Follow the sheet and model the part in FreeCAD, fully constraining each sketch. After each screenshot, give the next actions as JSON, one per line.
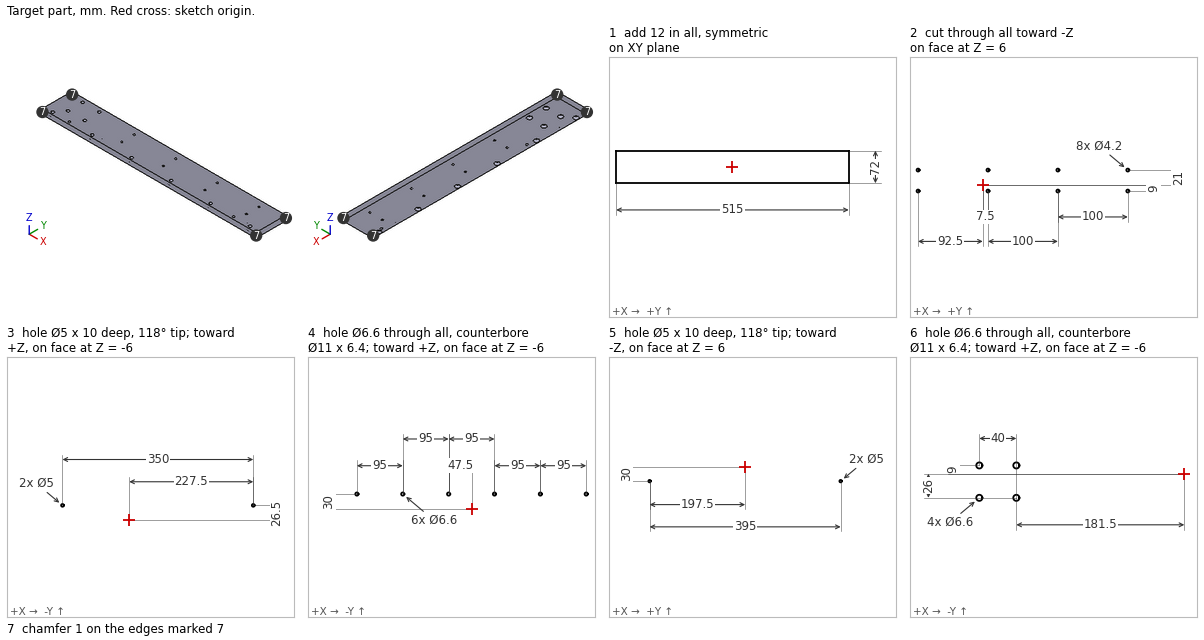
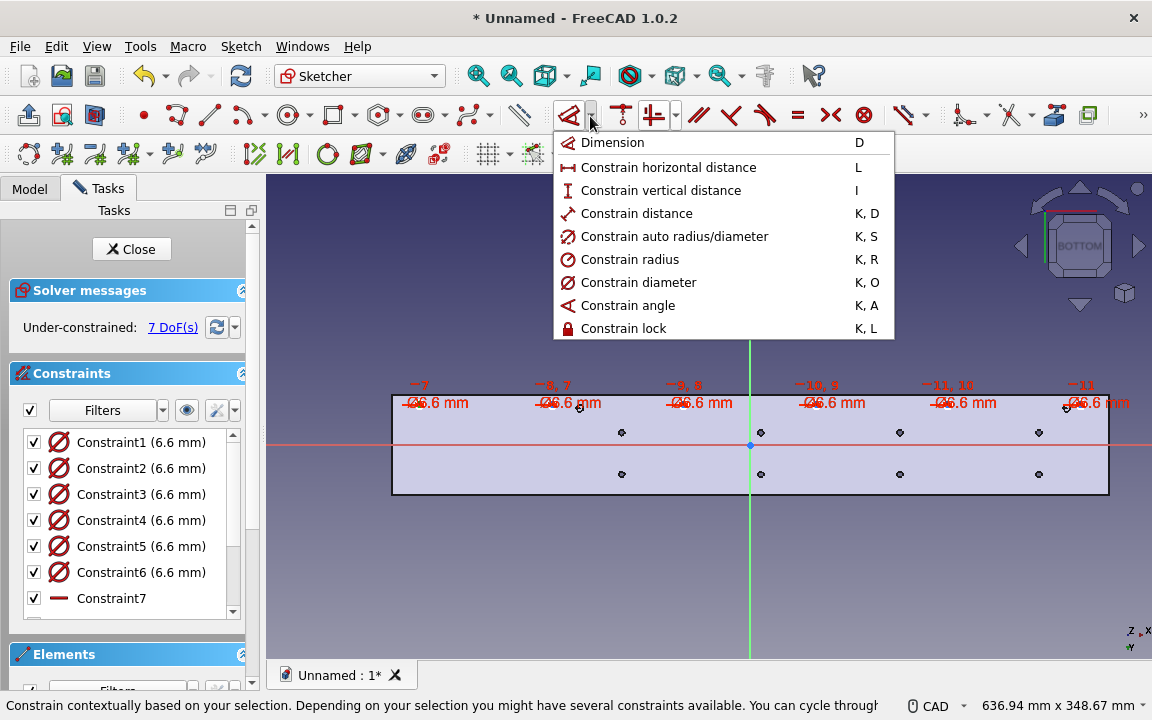
{"action": "left_click", "coordinate": [724, 190]}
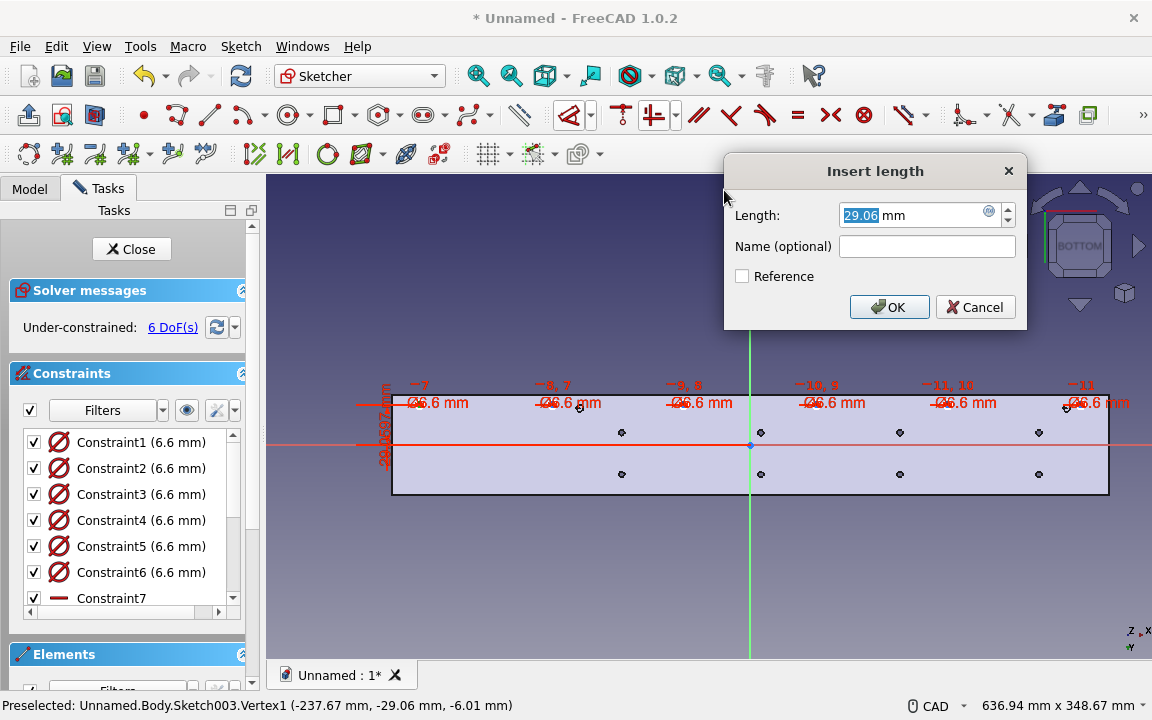
{"action": "type", "text": "30"}
{"action": "key", "text": "Return"}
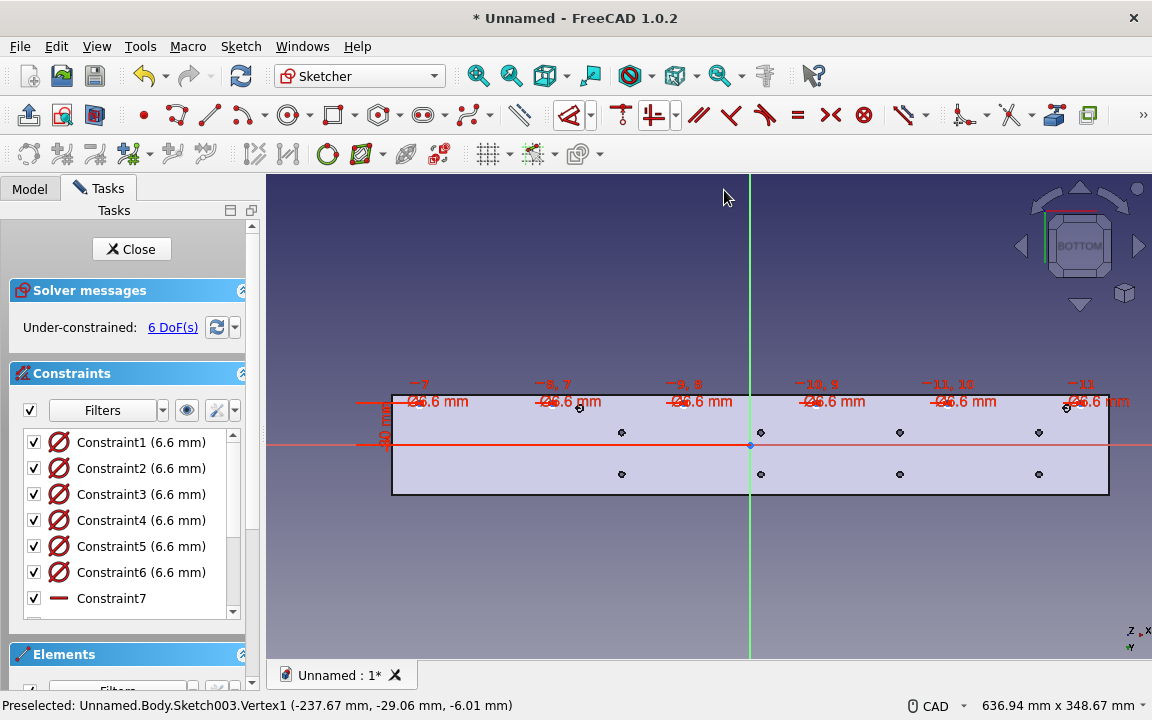
{"action": "left_click", "coordinate": [420, 403]}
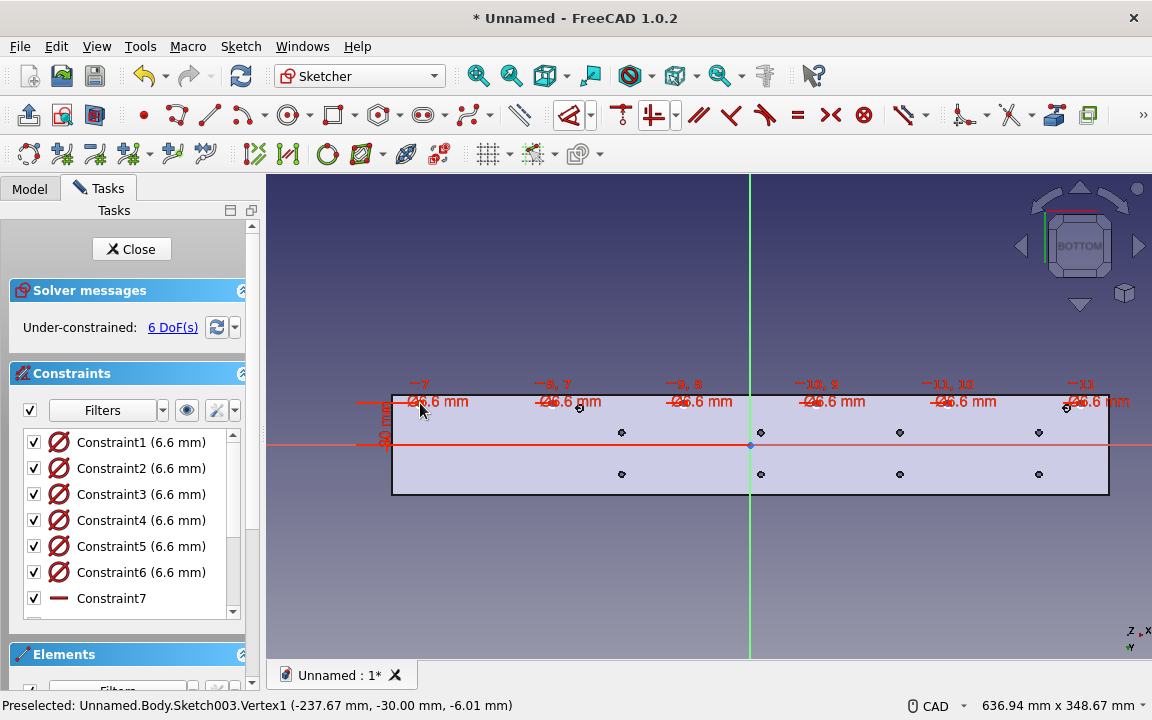
{"action": "left_click", "coordinate": [552, 403]}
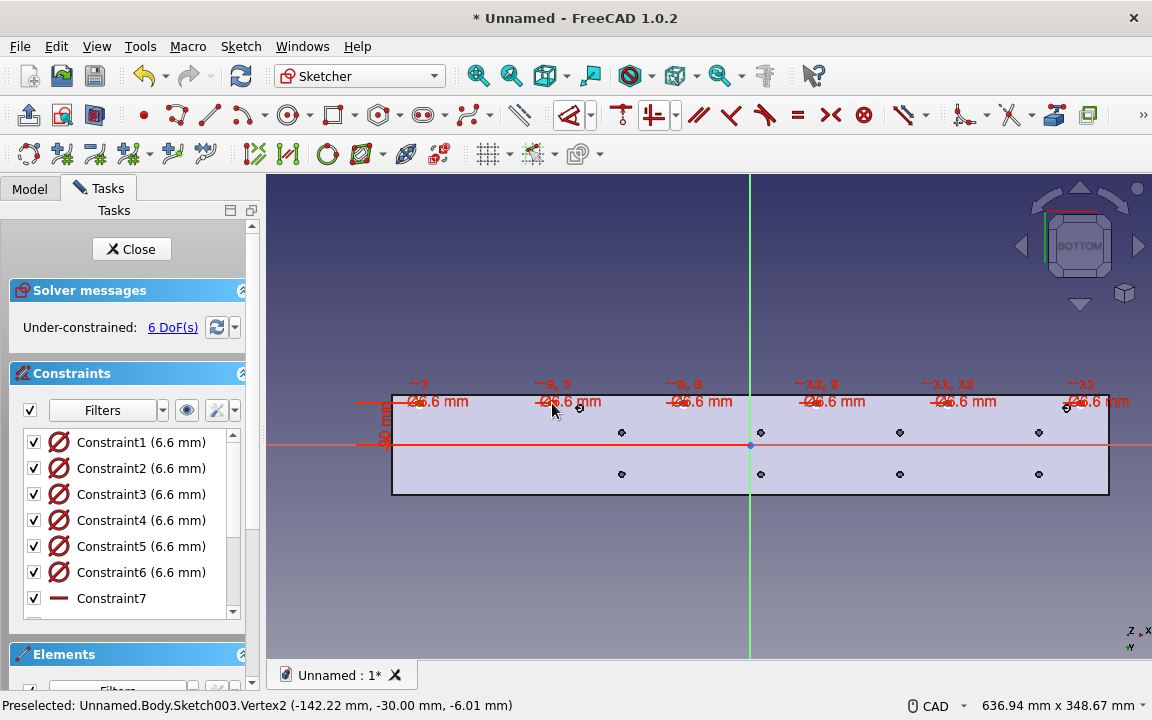
{"action": "key", "text": "l"}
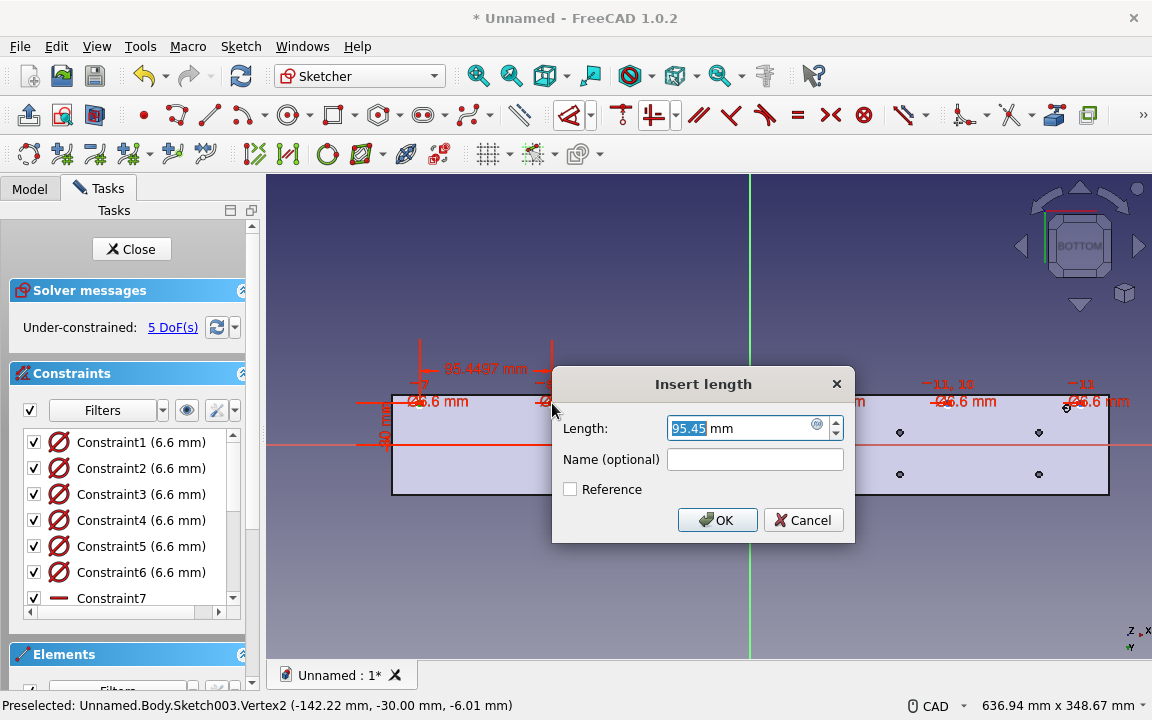
{"action": "type", "text": "95"}
{"action": "key", "text": "Return"}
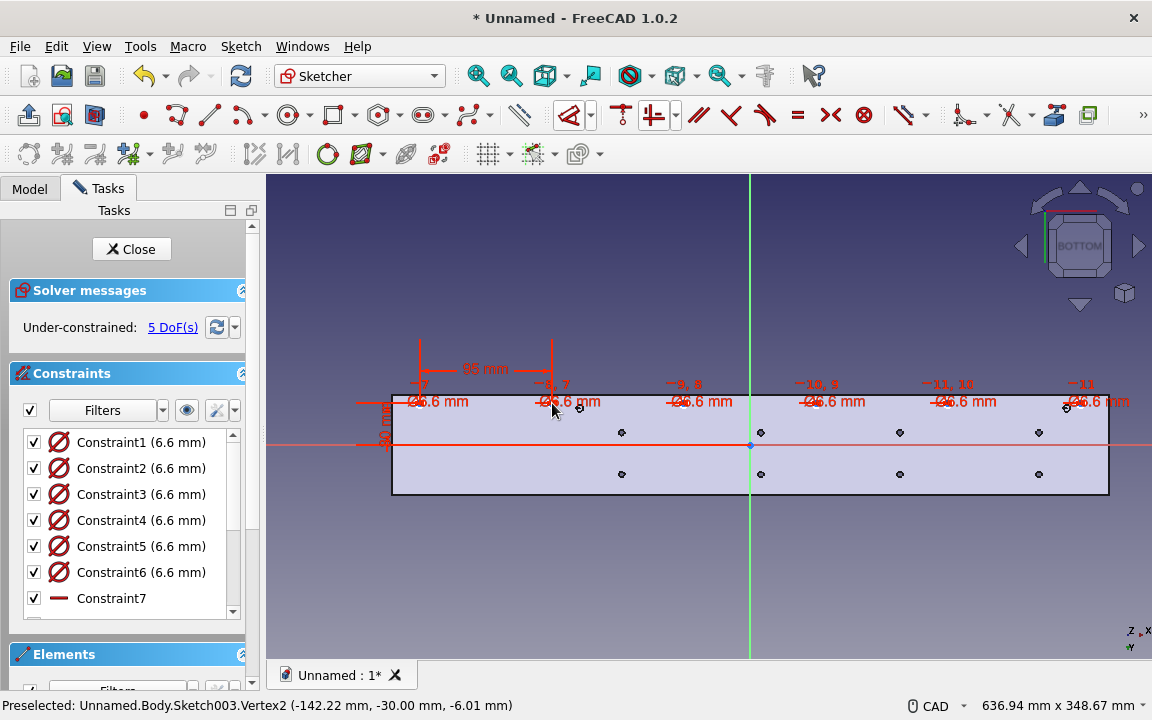
{"action": "left_click", "coordinate": [552, 403]}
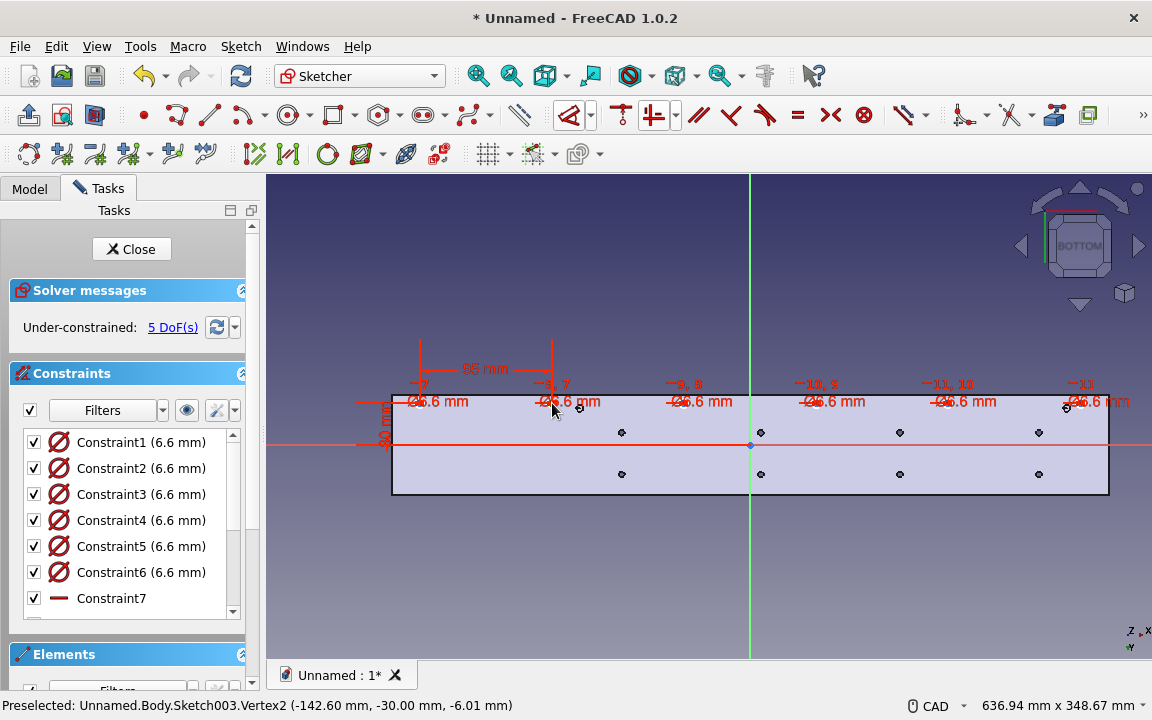
{"action": "left_click", "coordinate": [684, 403]}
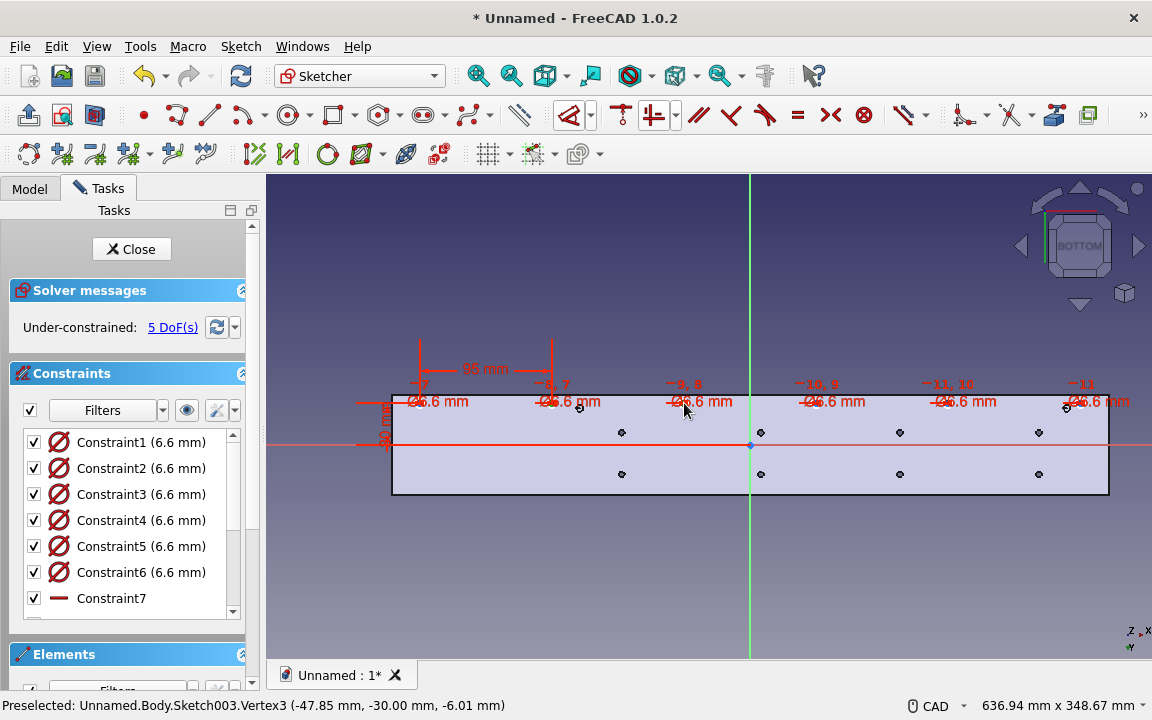
{"action": "key", "text": "l"}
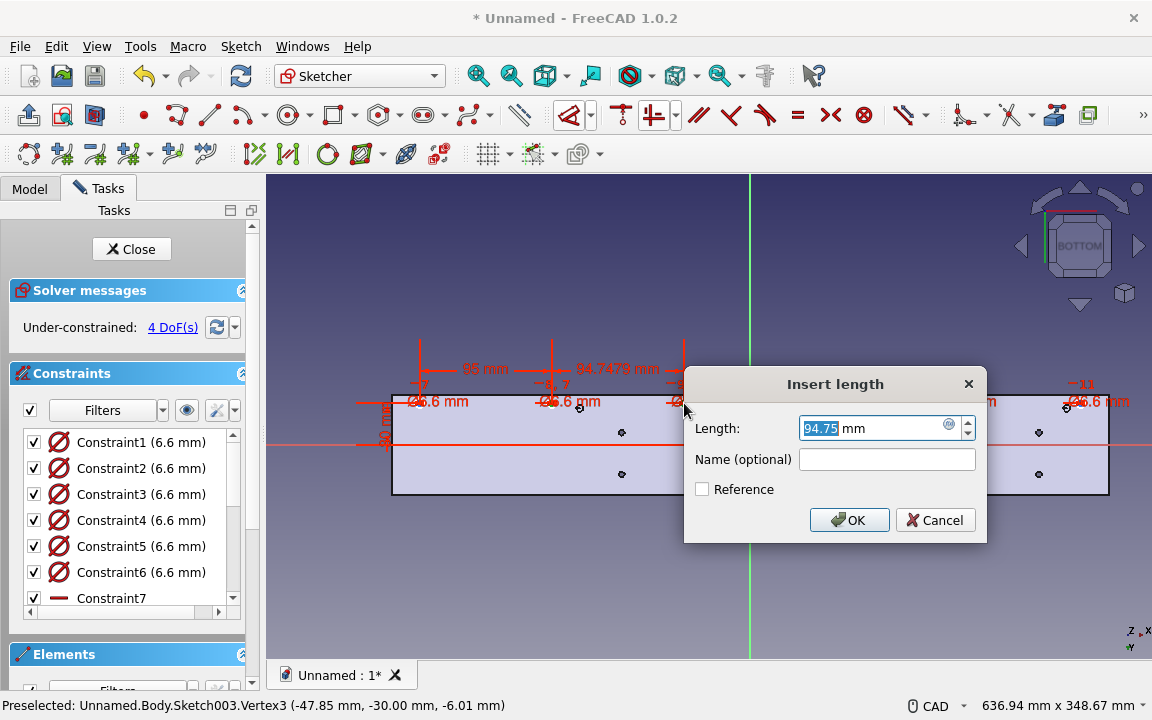
{"action": "type", "text": "95"}
{"action": "key", "text": "Return"}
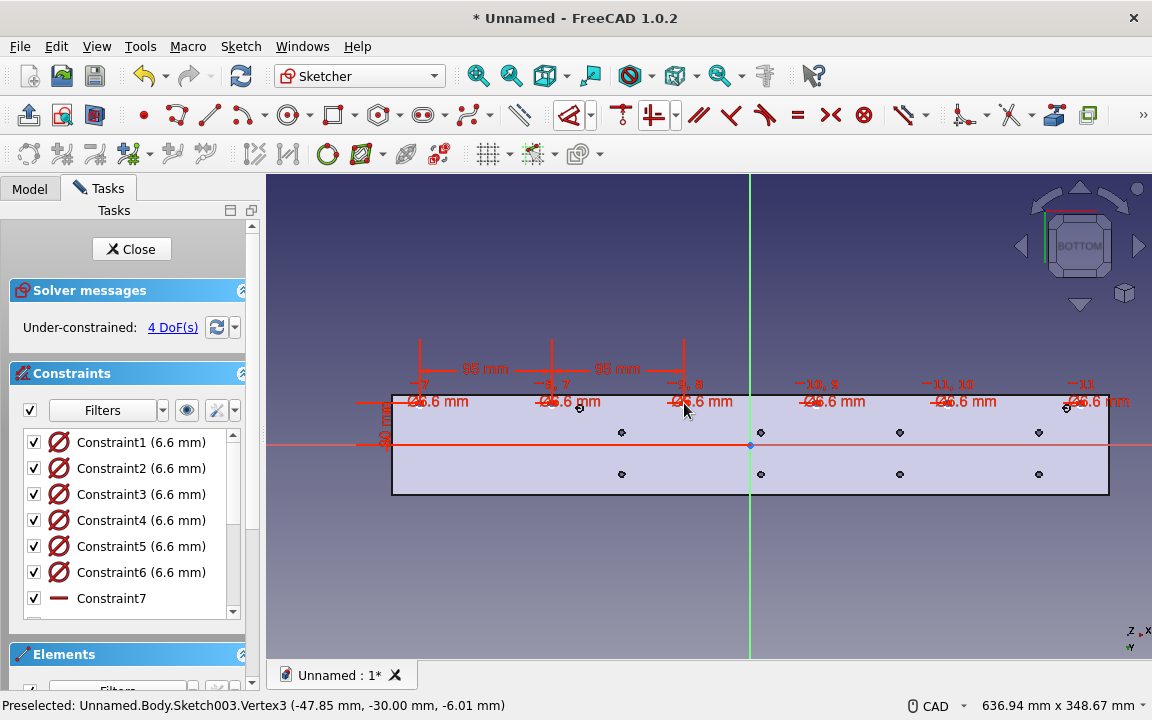
{"action": "left_click", "coordinate": [684, 403]}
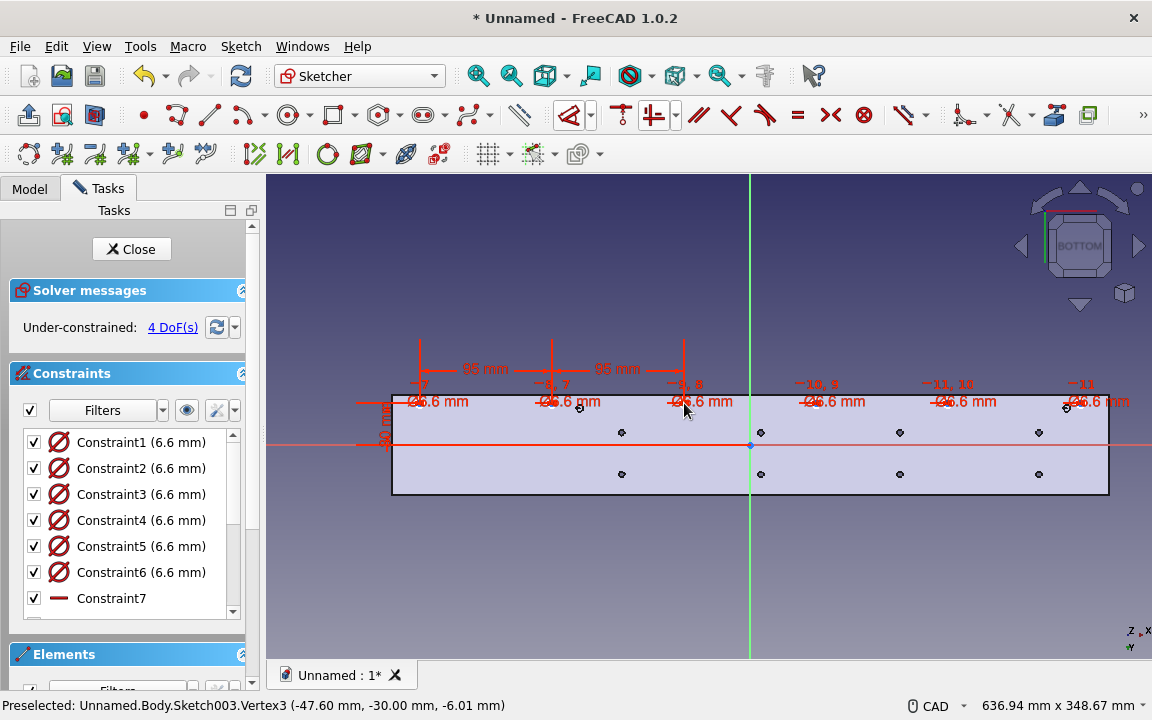
{"action": "left_click", "coordinate": [817, 403]}